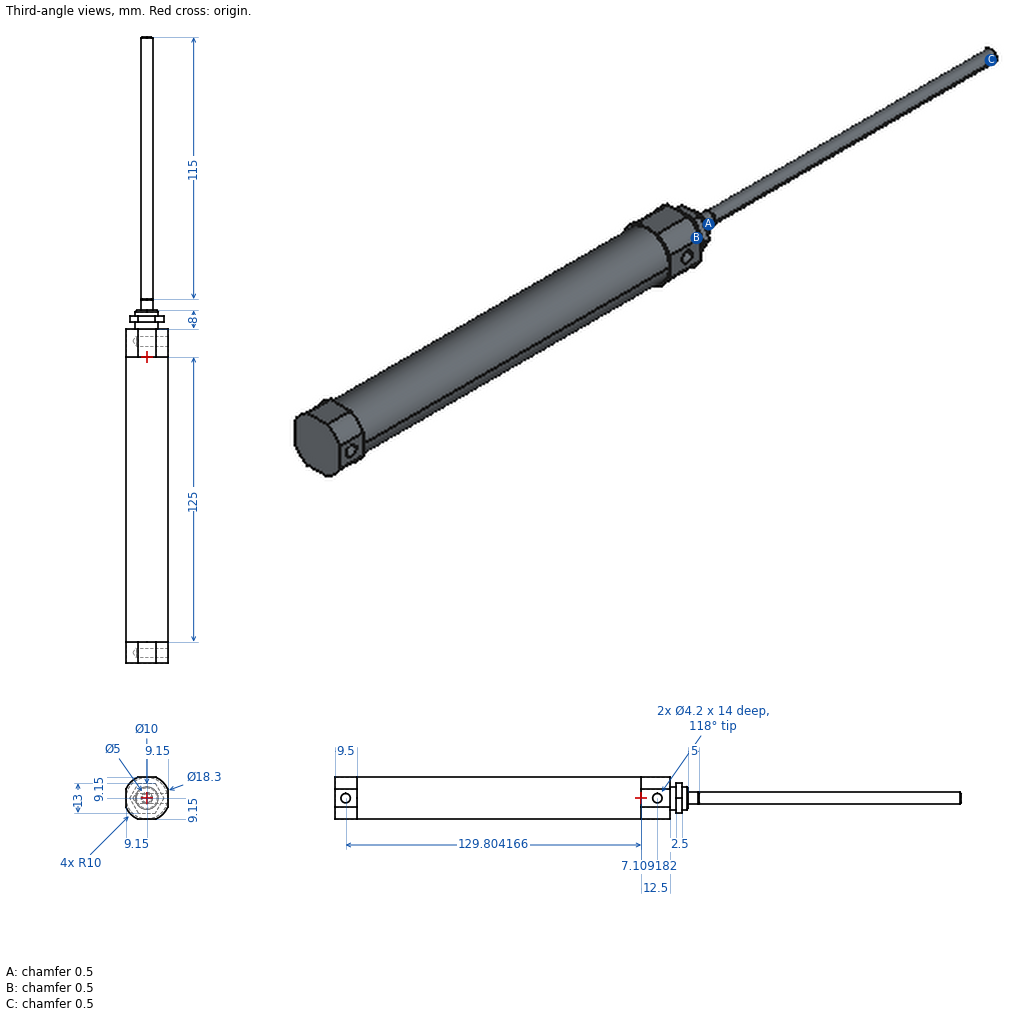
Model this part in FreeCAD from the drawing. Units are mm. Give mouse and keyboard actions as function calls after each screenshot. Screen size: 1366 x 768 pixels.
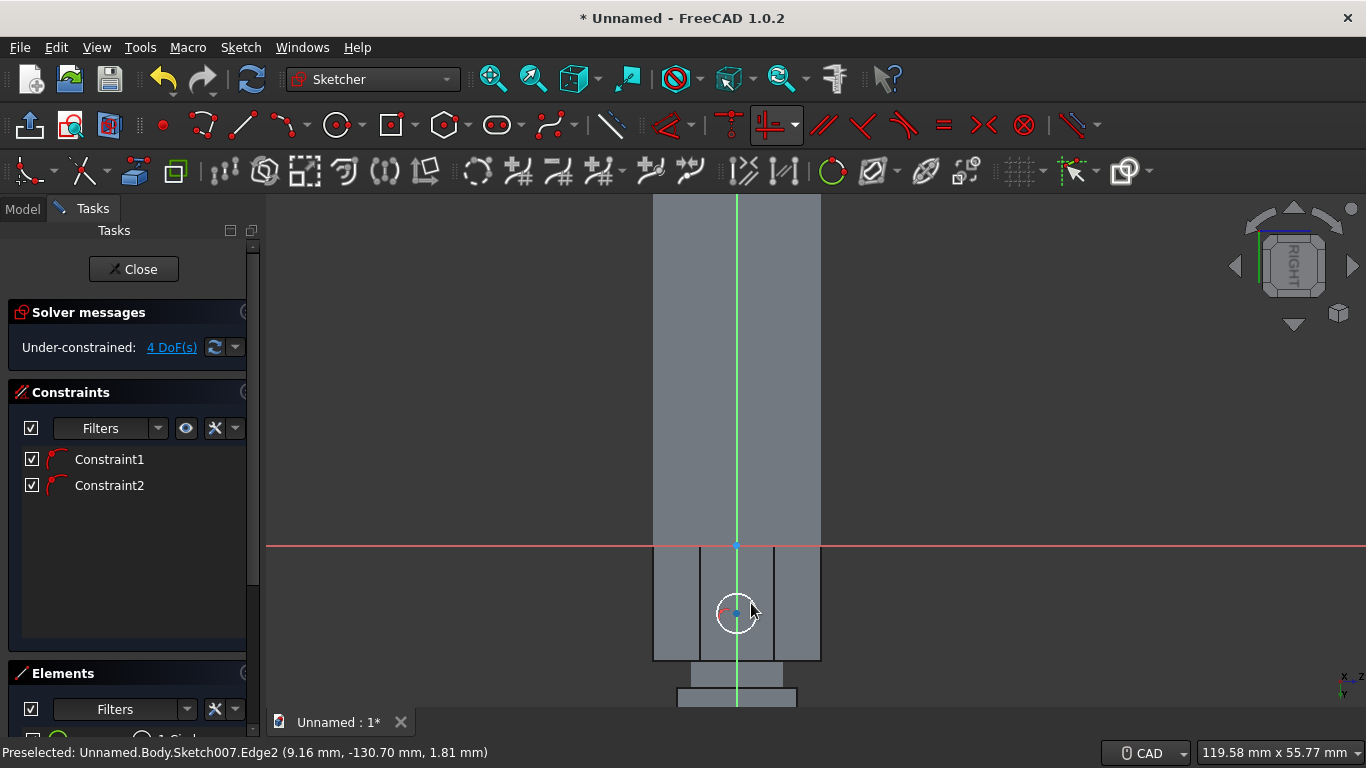
click(751, 600)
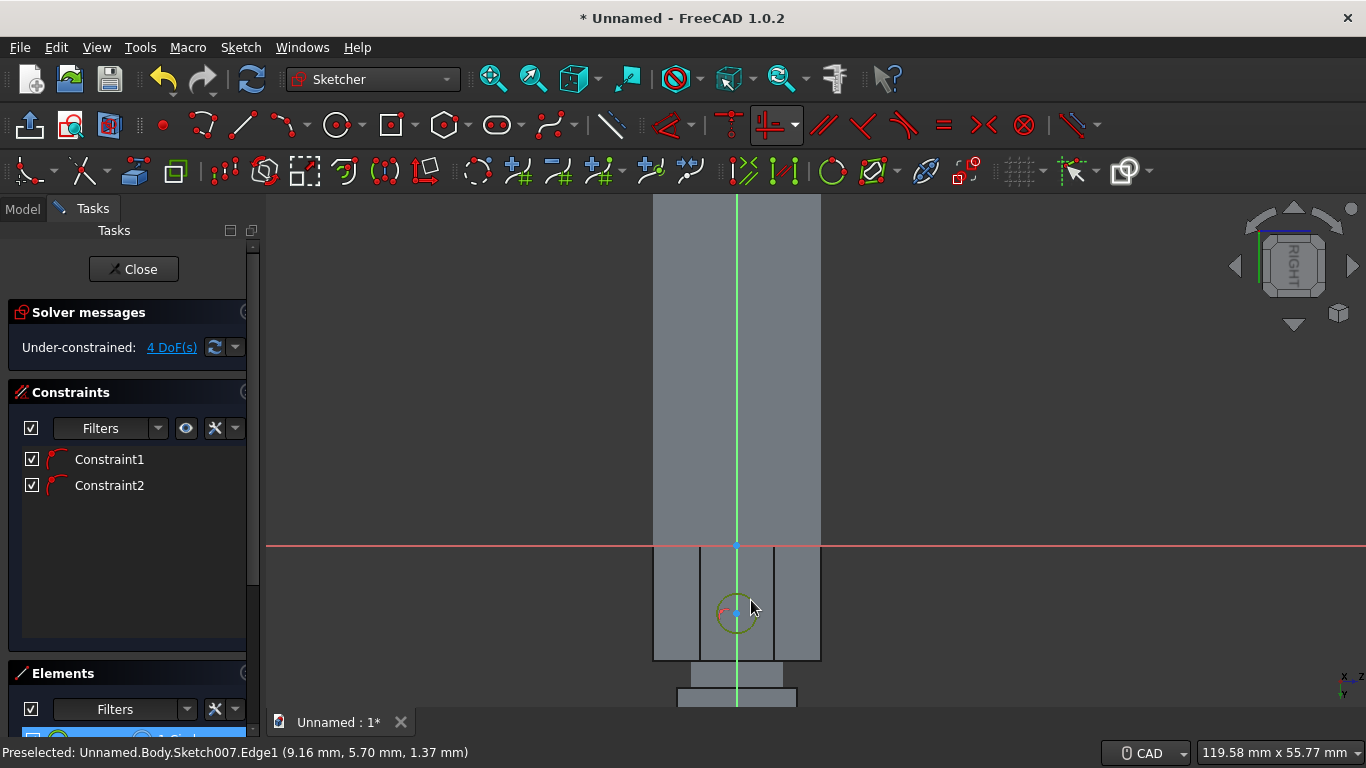
scroll(751, 604, down, 7)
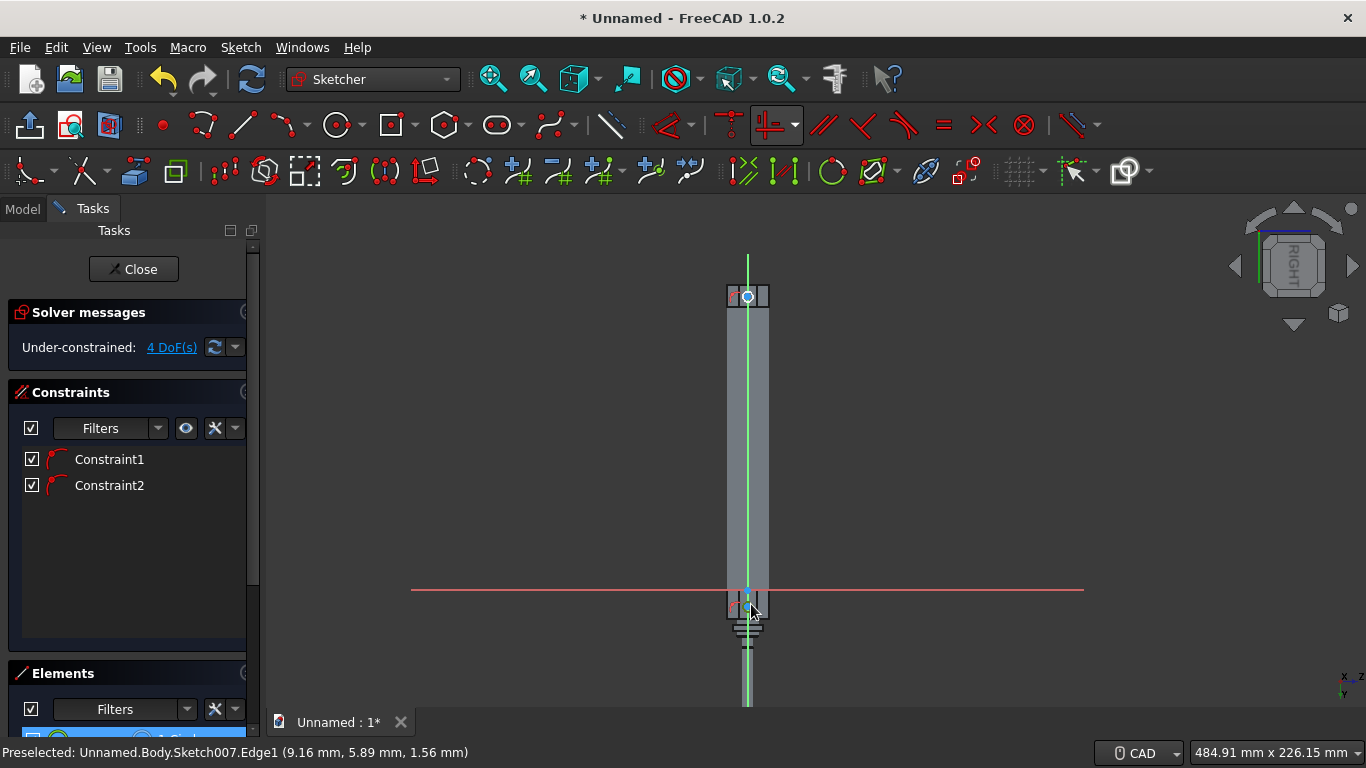
scroll(751, 293, up, 7)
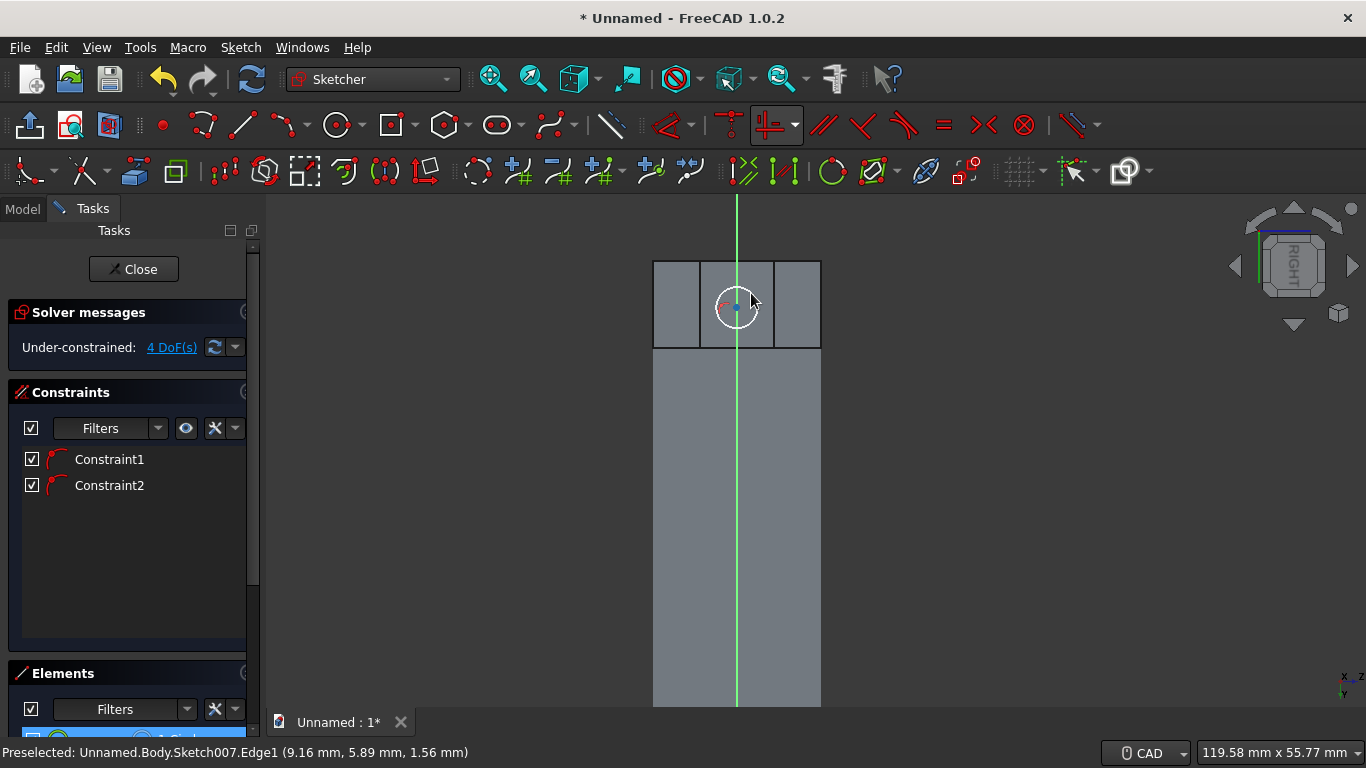
click(751, 293)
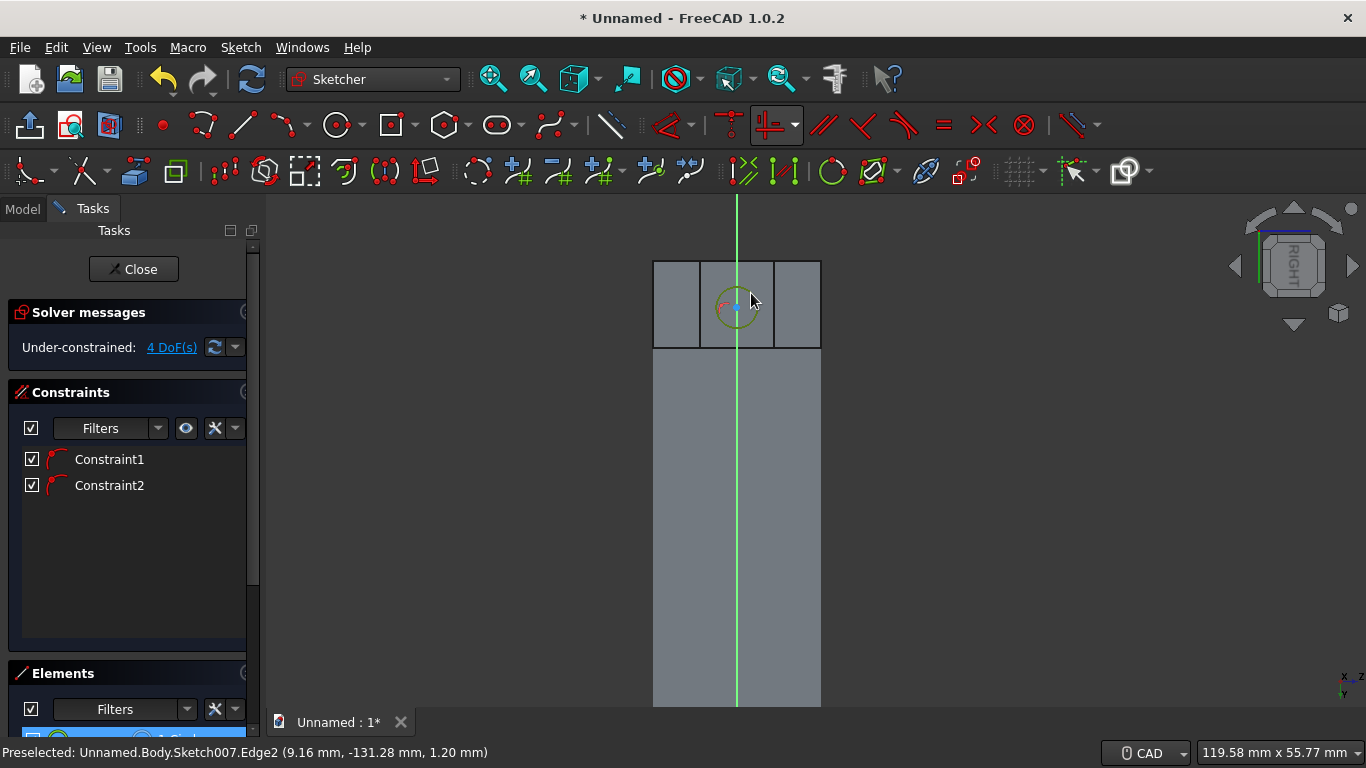
key(e)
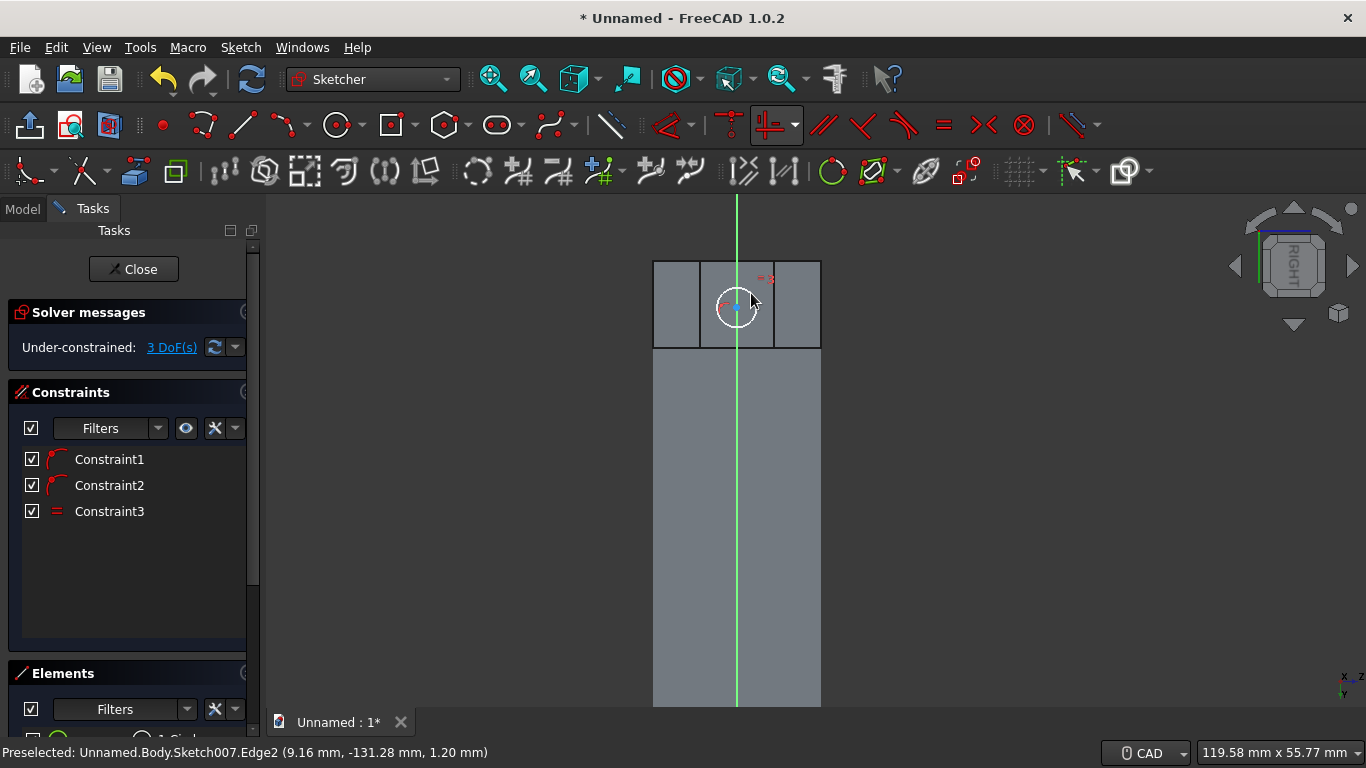
click(666, 126)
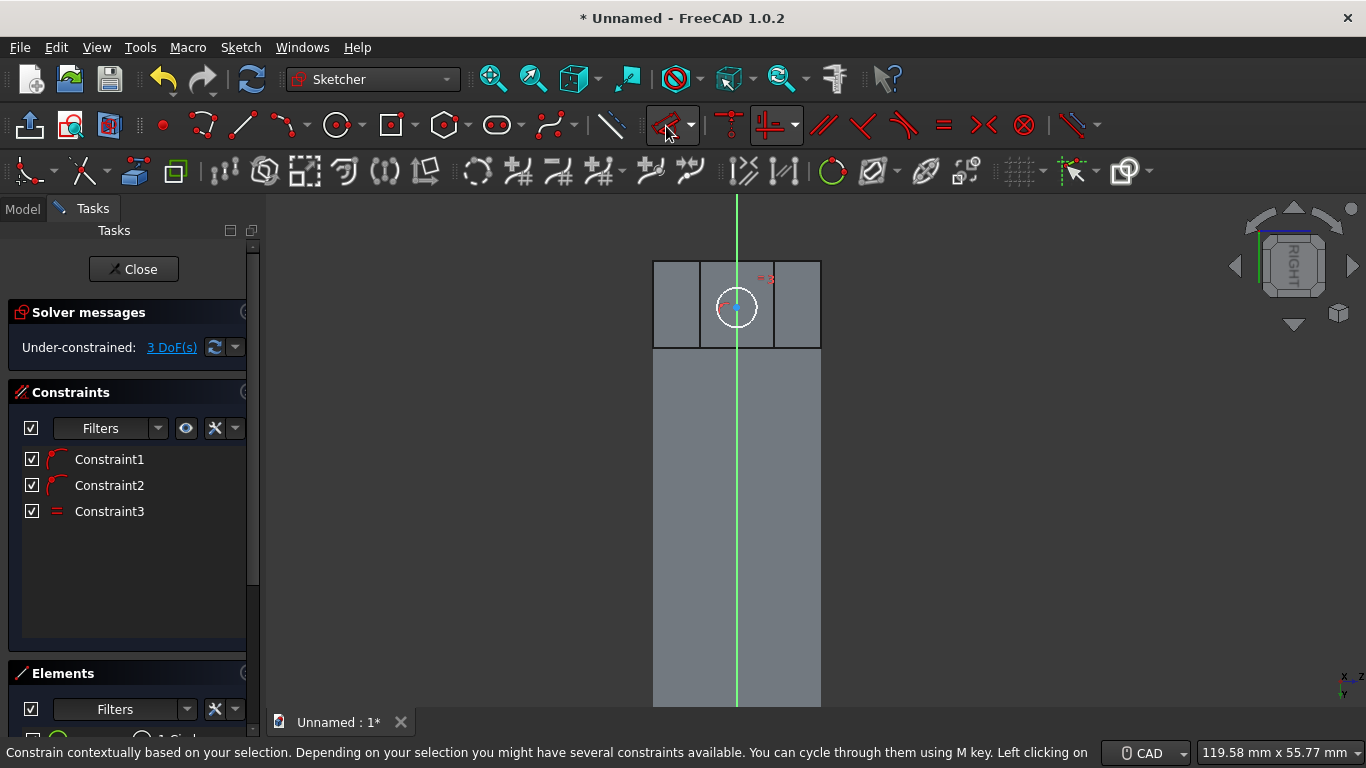
scroll(751, 292, down, 7)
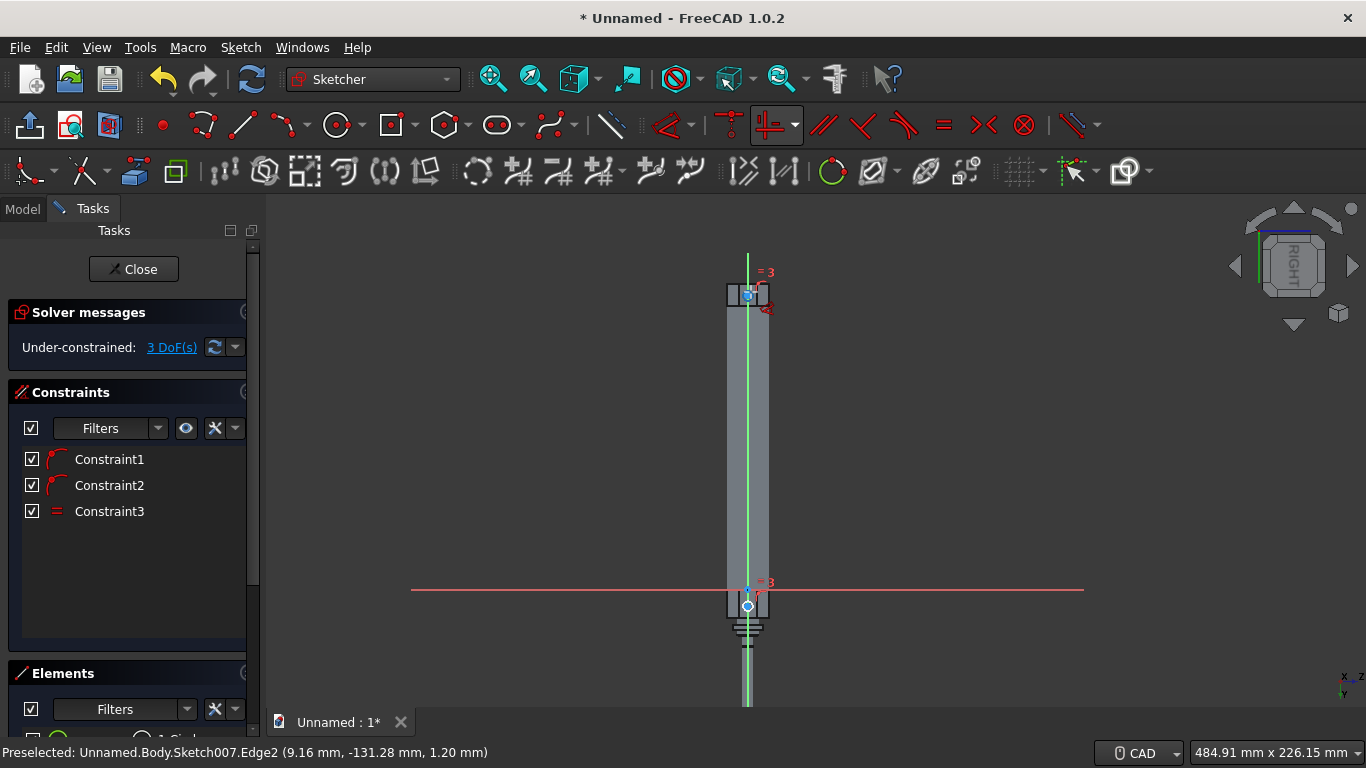
scroll(751, 603, up, 8)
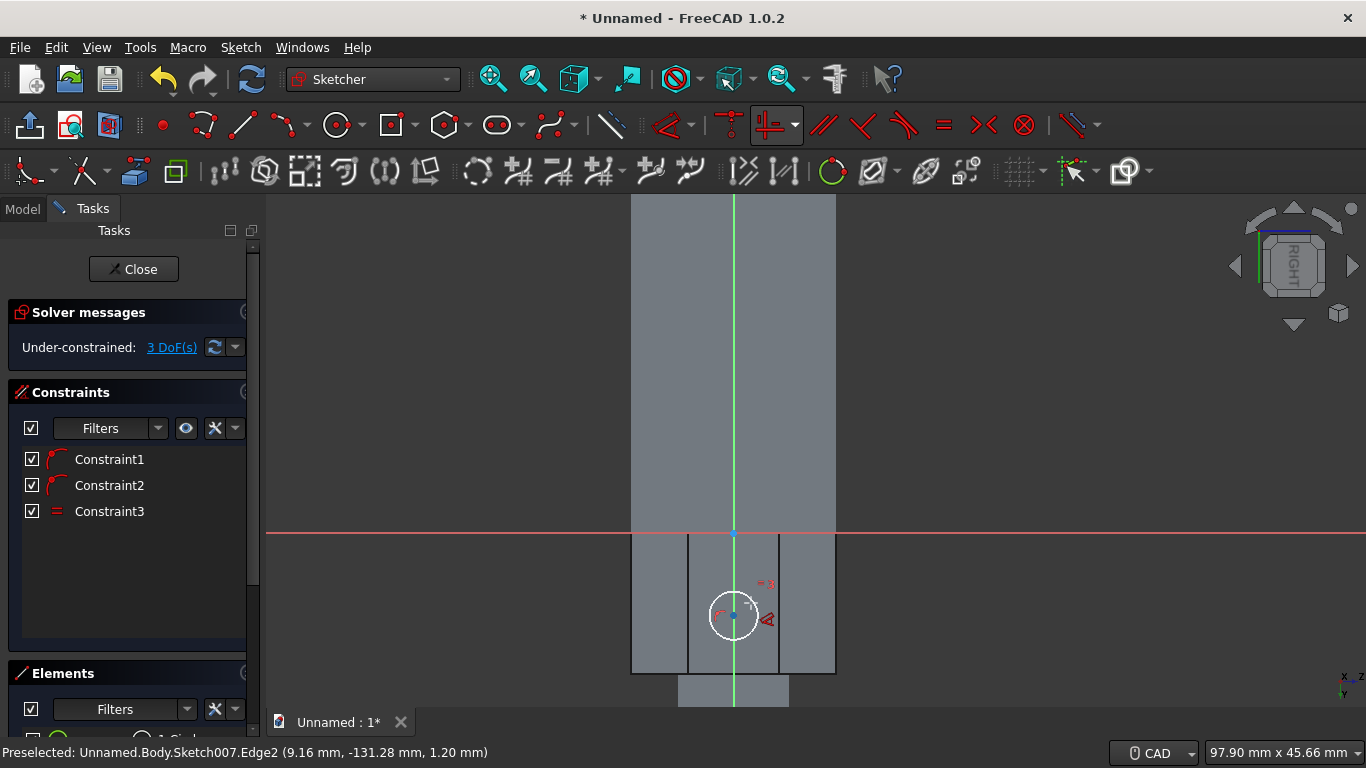
click(751, 599)
click(774, 577)